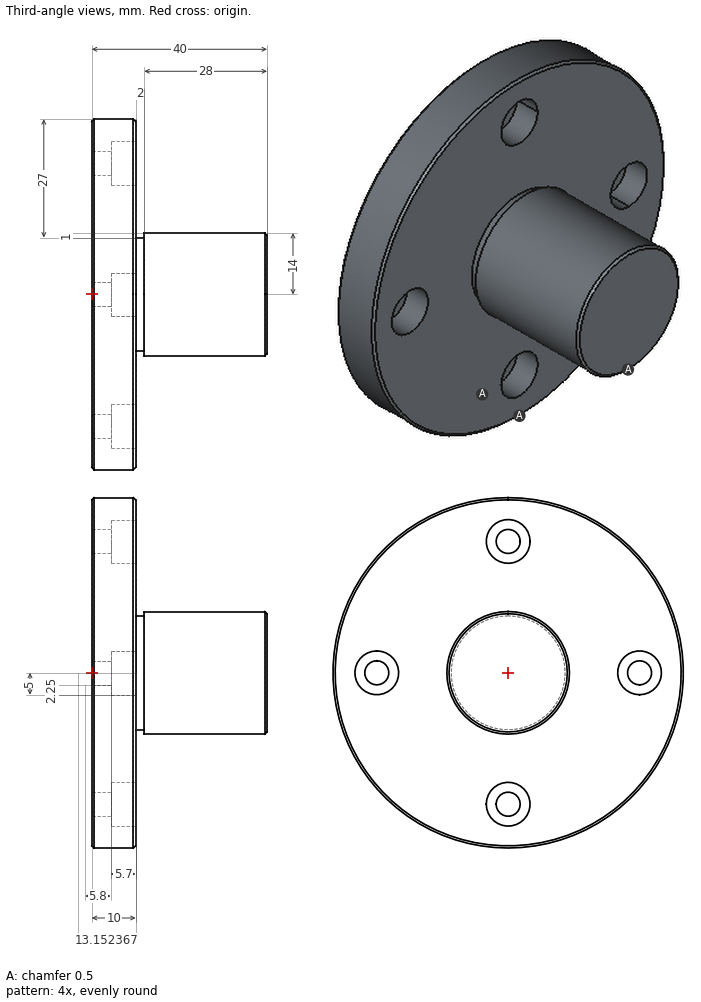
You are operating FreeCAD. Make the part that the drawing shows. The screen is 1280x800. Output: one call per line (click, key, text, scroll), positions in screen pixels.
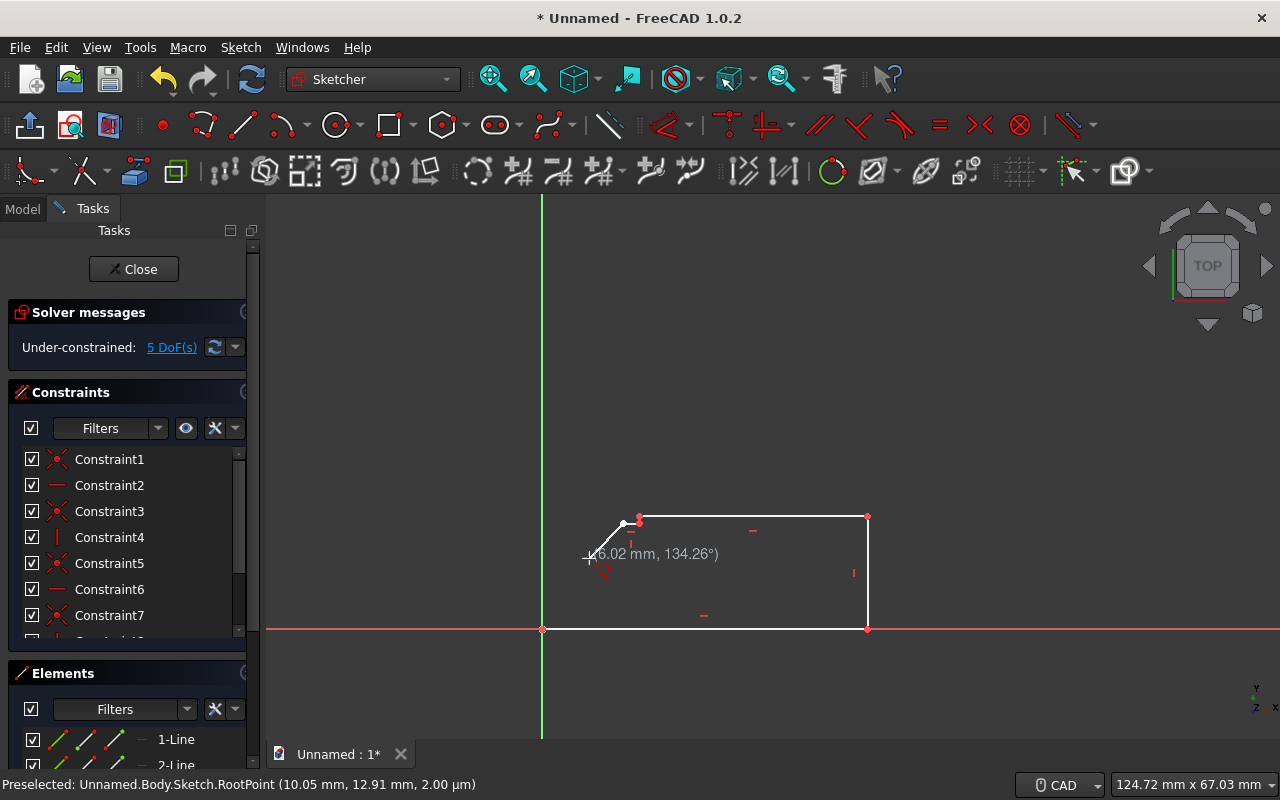
click(623, 304)
click(551, 304)
click(542, 629)
key(Escape)
key(Escape)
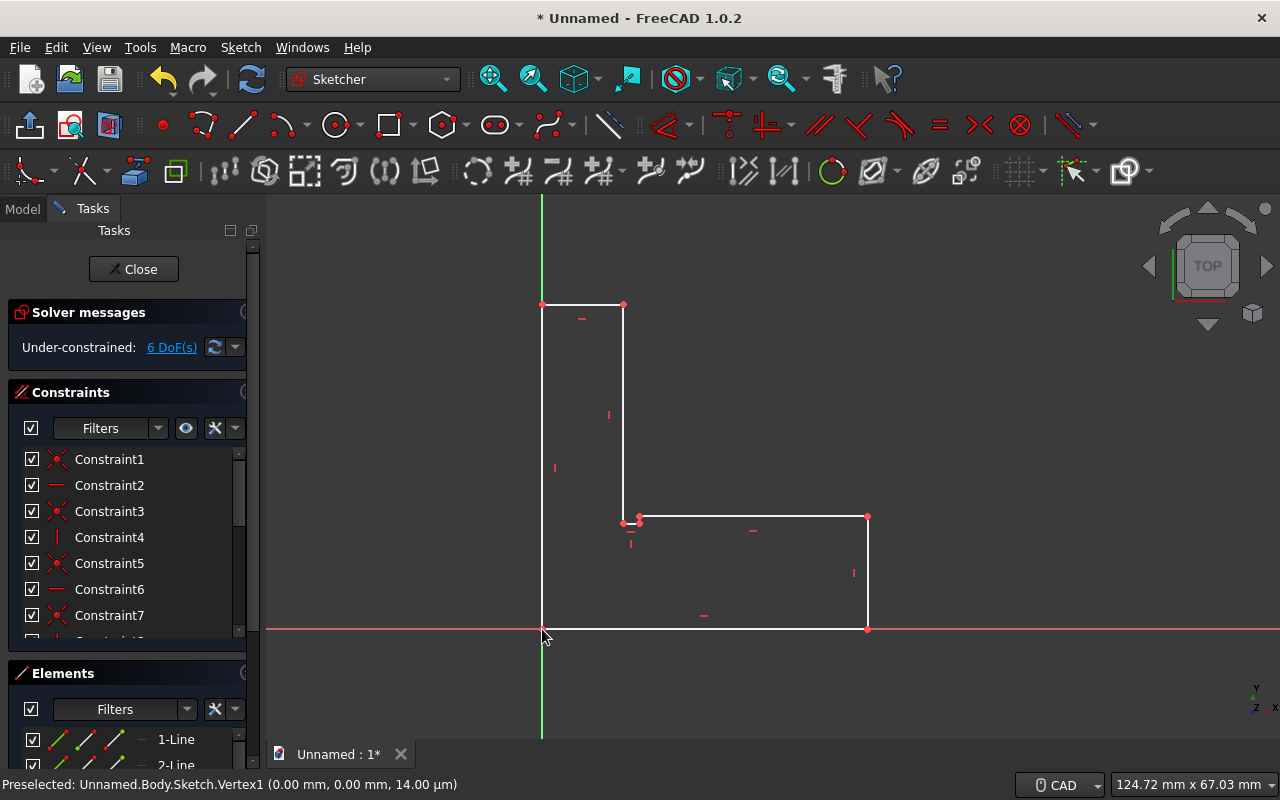
scroll(640, 520, up, 8)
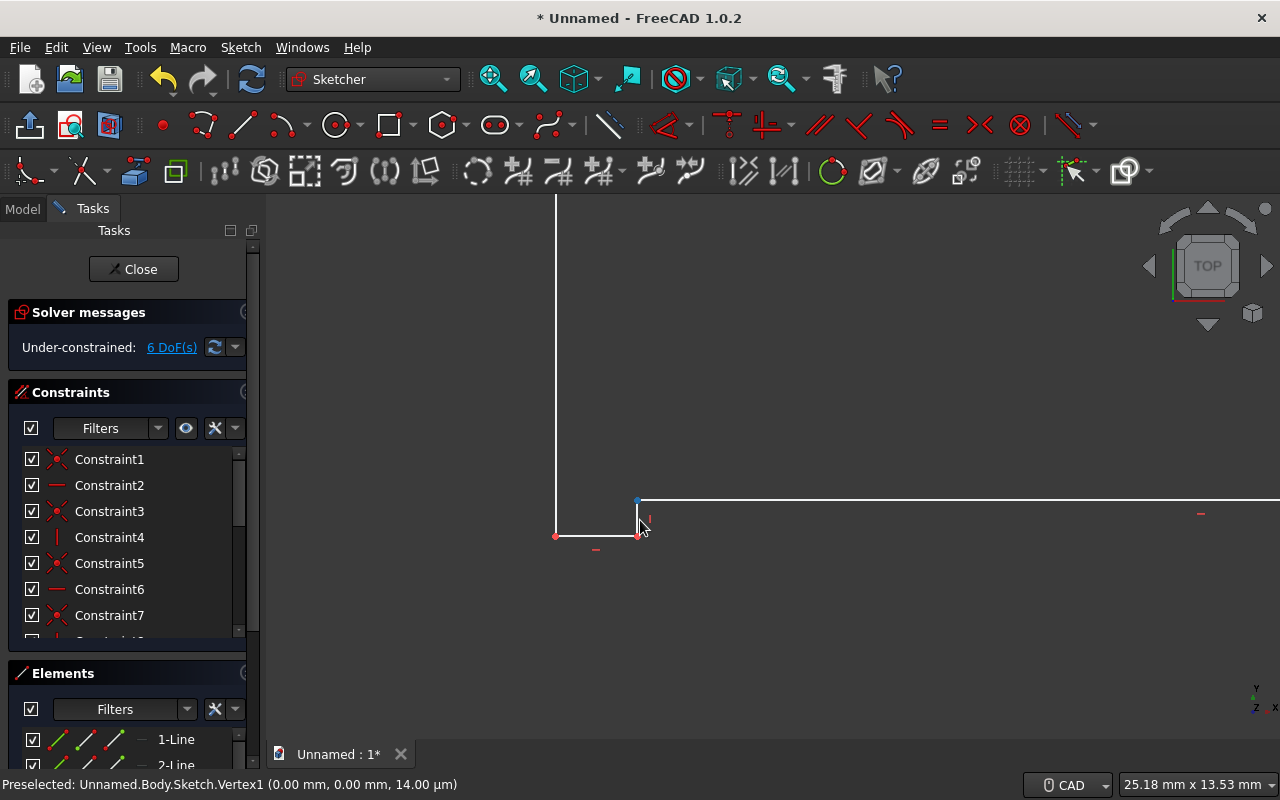
click(637, 518)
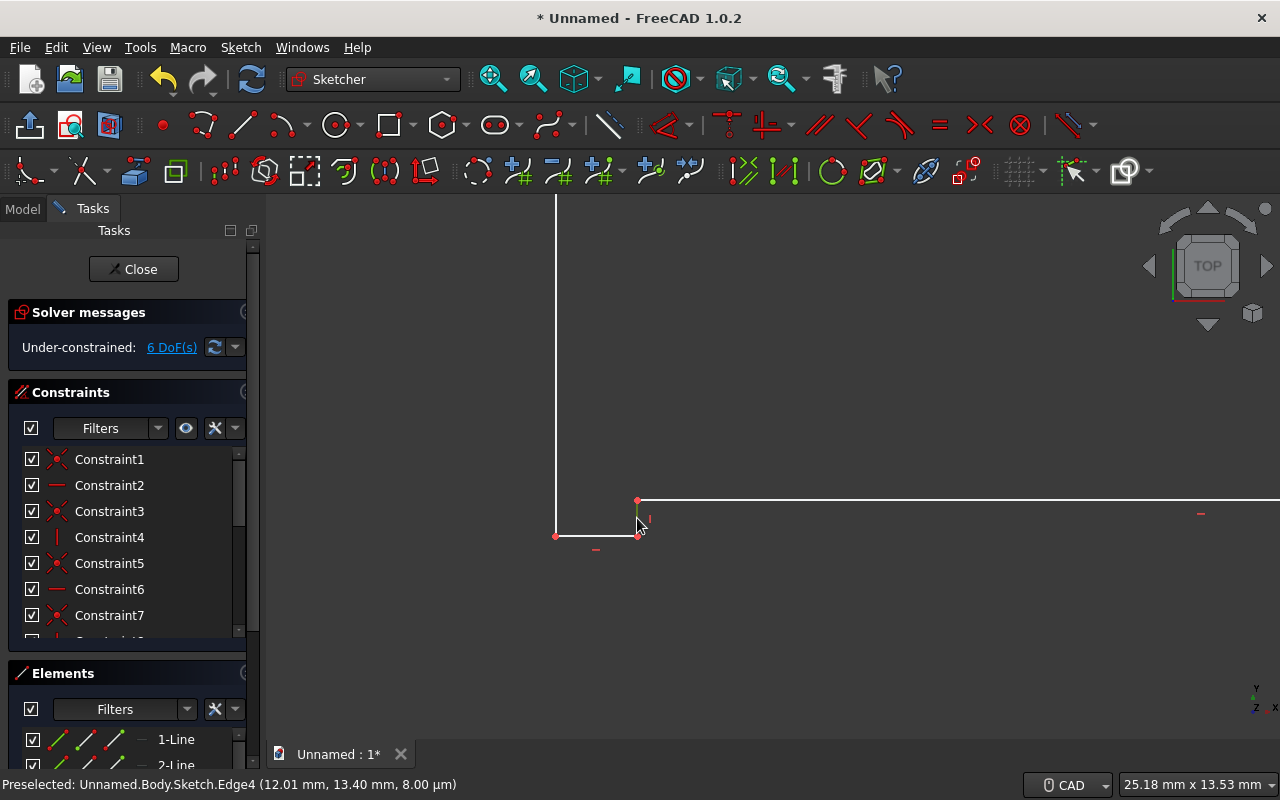
click(692, 126)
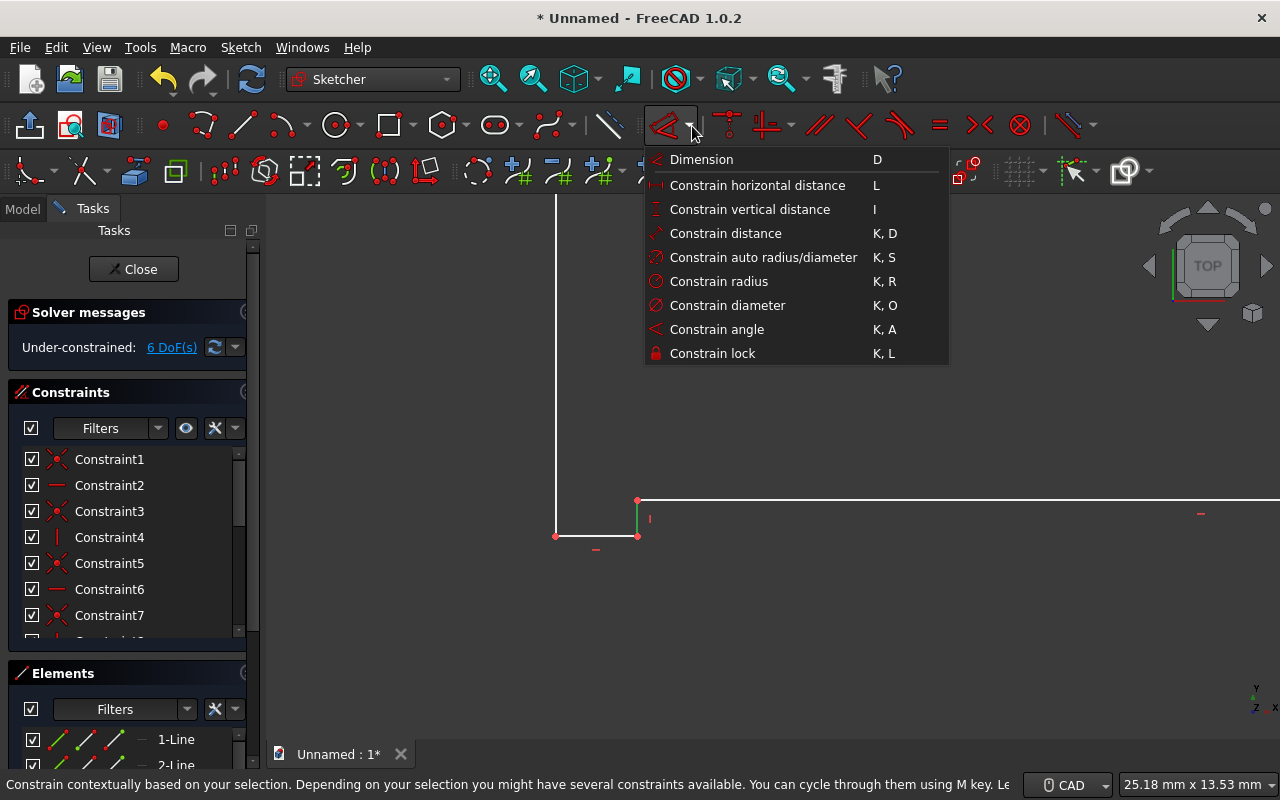
click(797, 209)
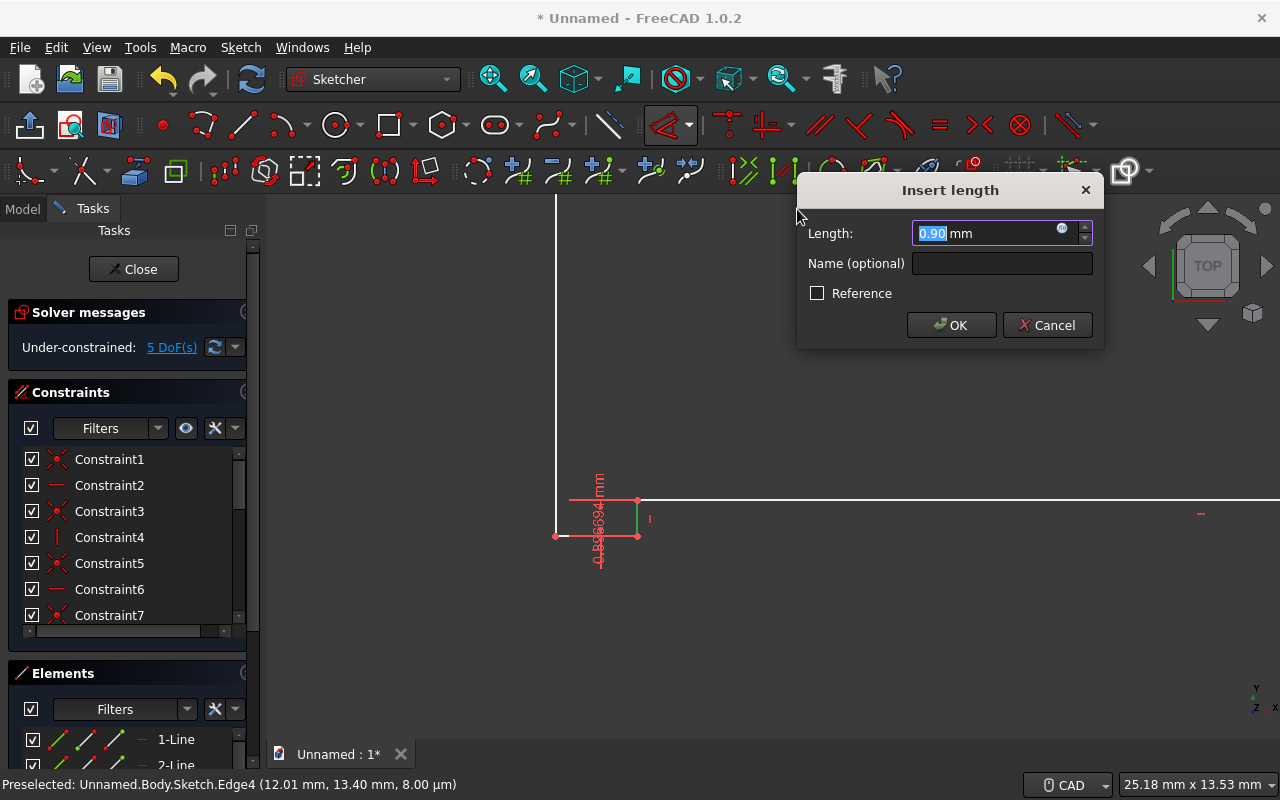
text(1)
key(Return)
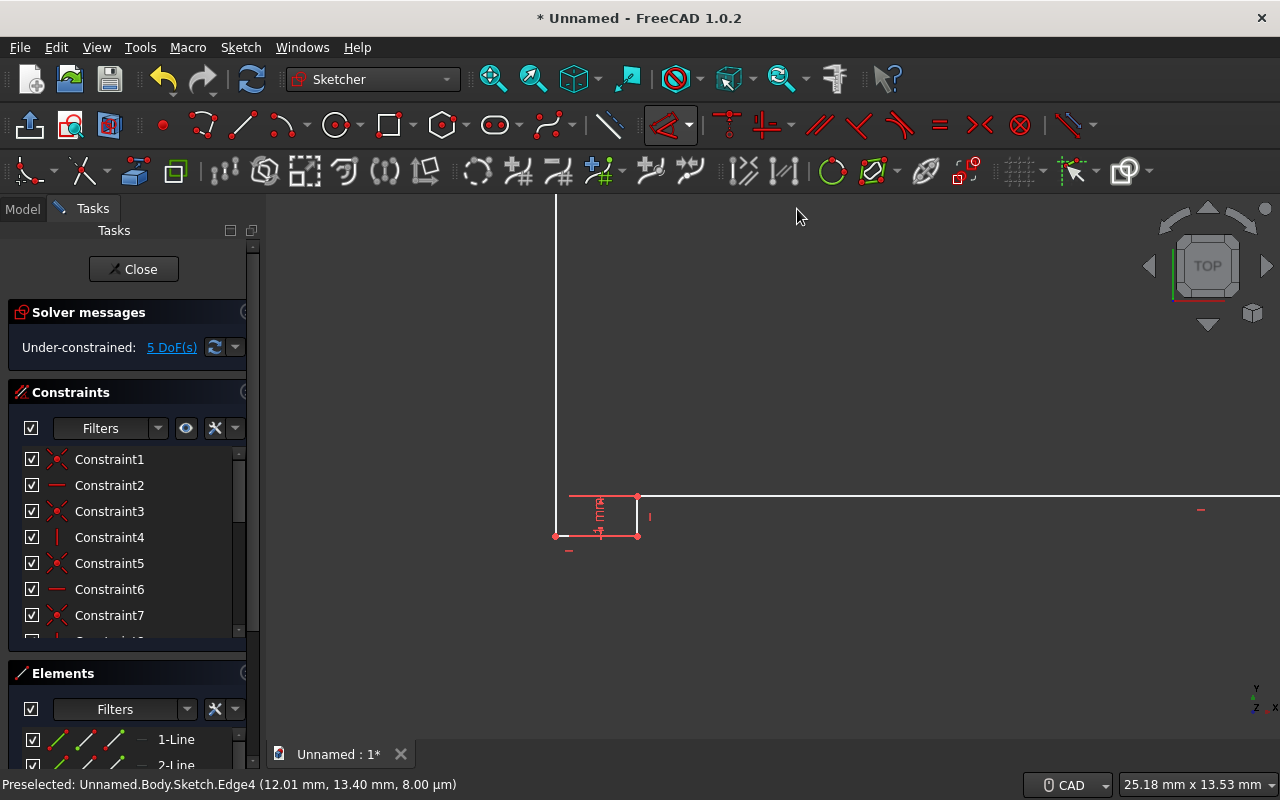
click(613, 536)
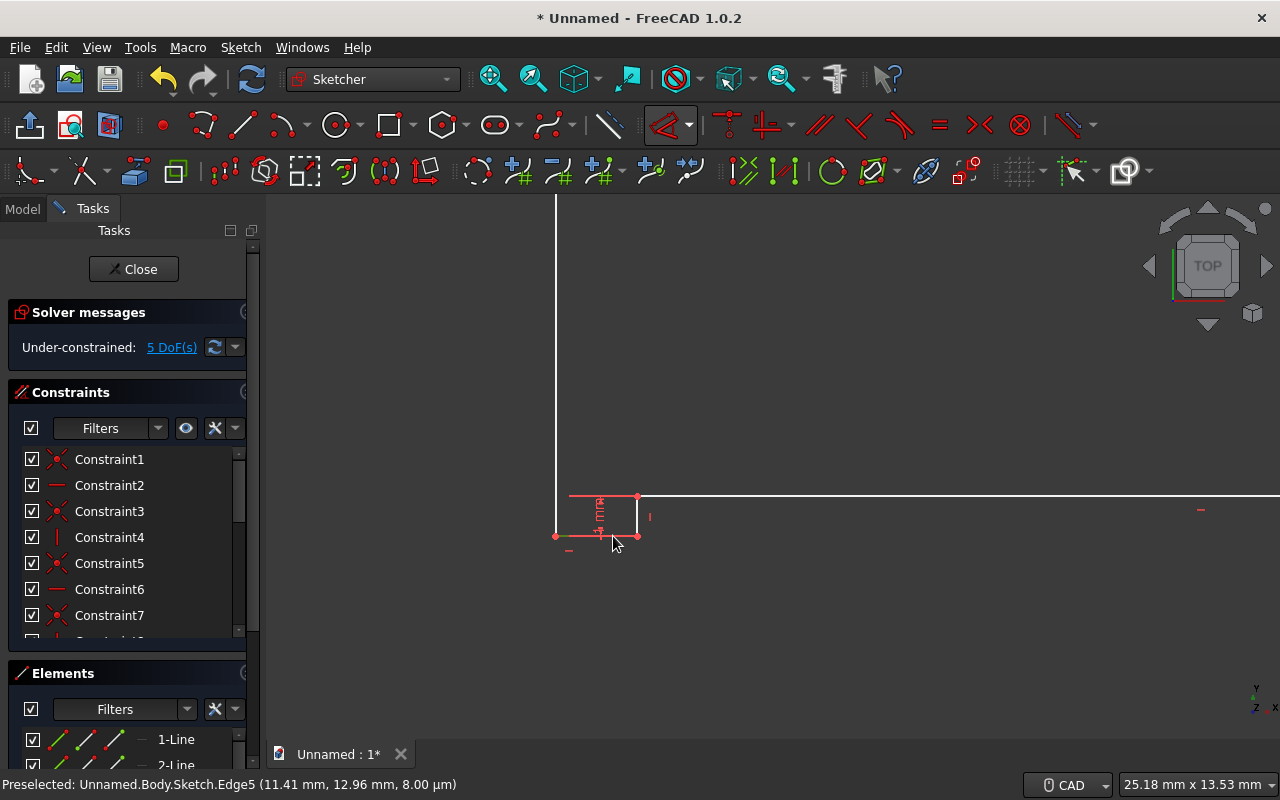
click(692, 126)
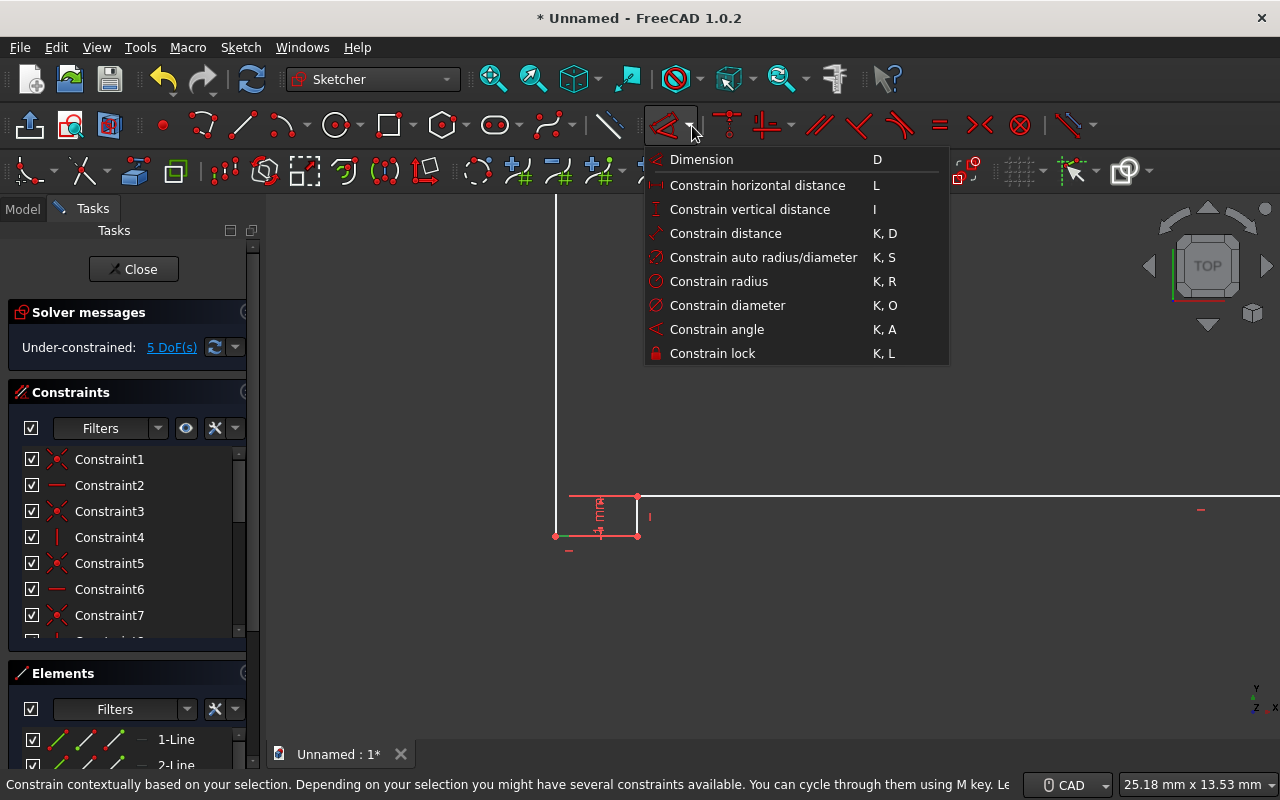
click(797, 185)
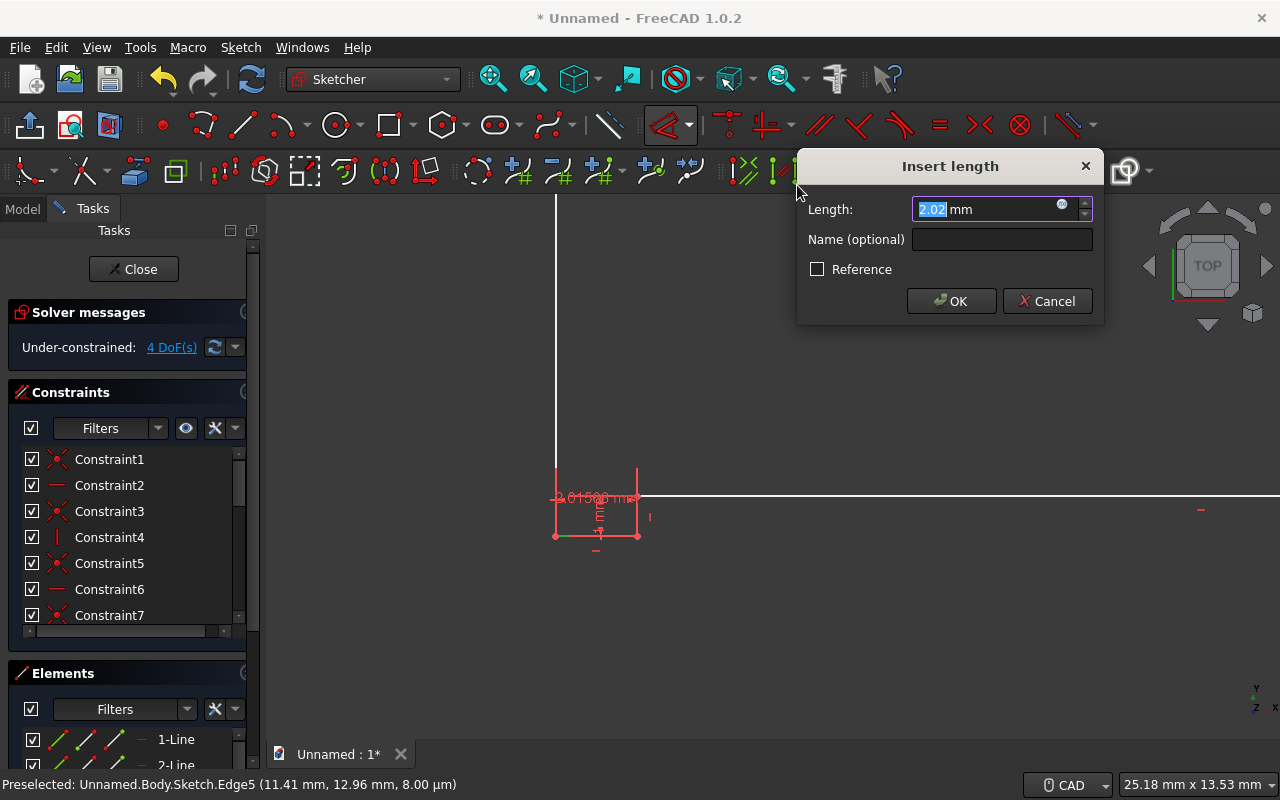
text(2)
key(Return)